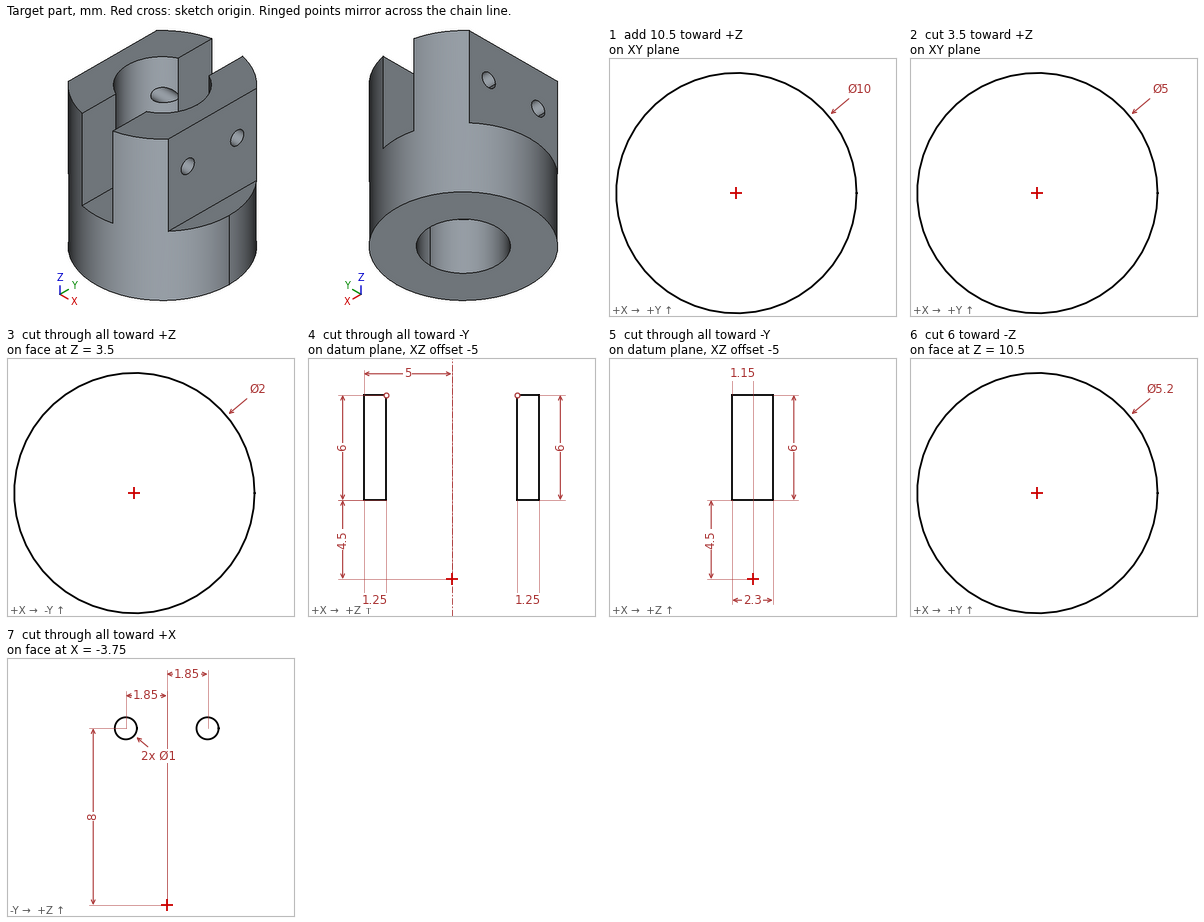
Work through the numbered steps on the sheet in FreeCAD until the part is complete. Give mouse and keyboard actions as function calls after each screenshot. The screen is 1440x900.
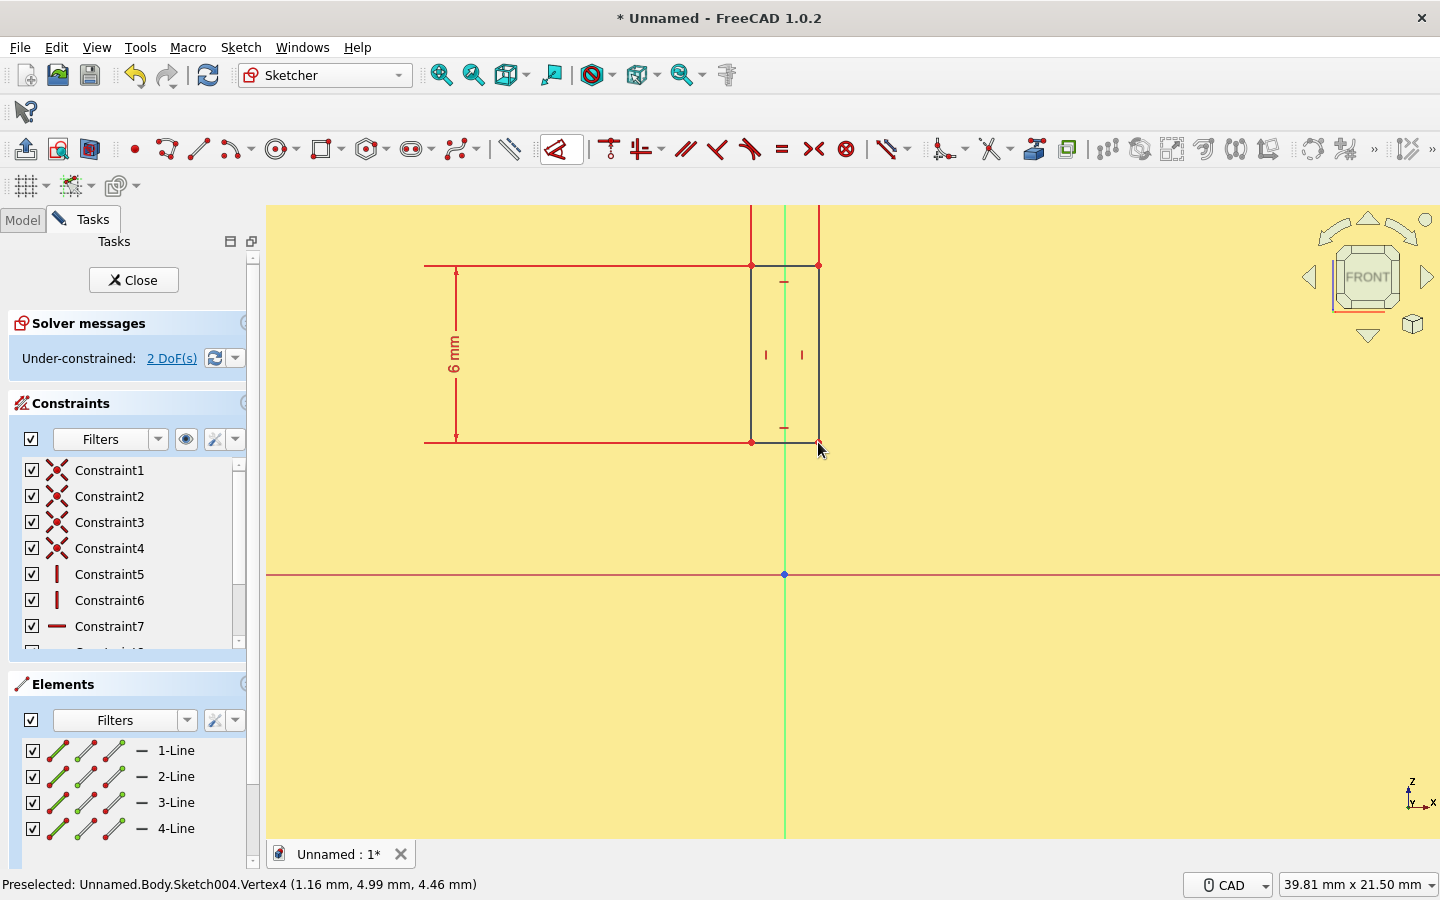
click(751, 443)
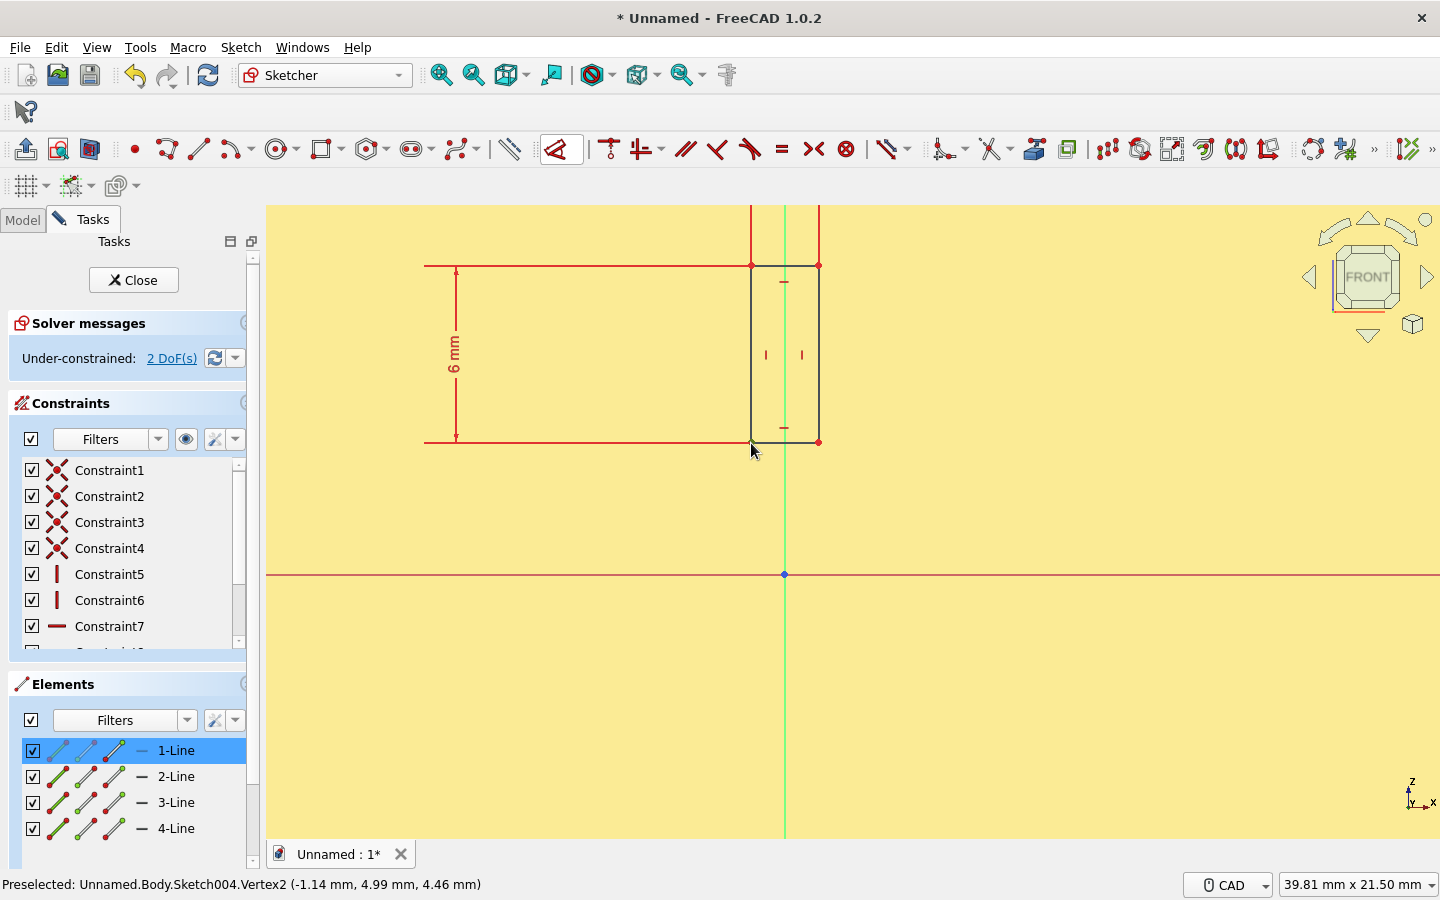
key(i)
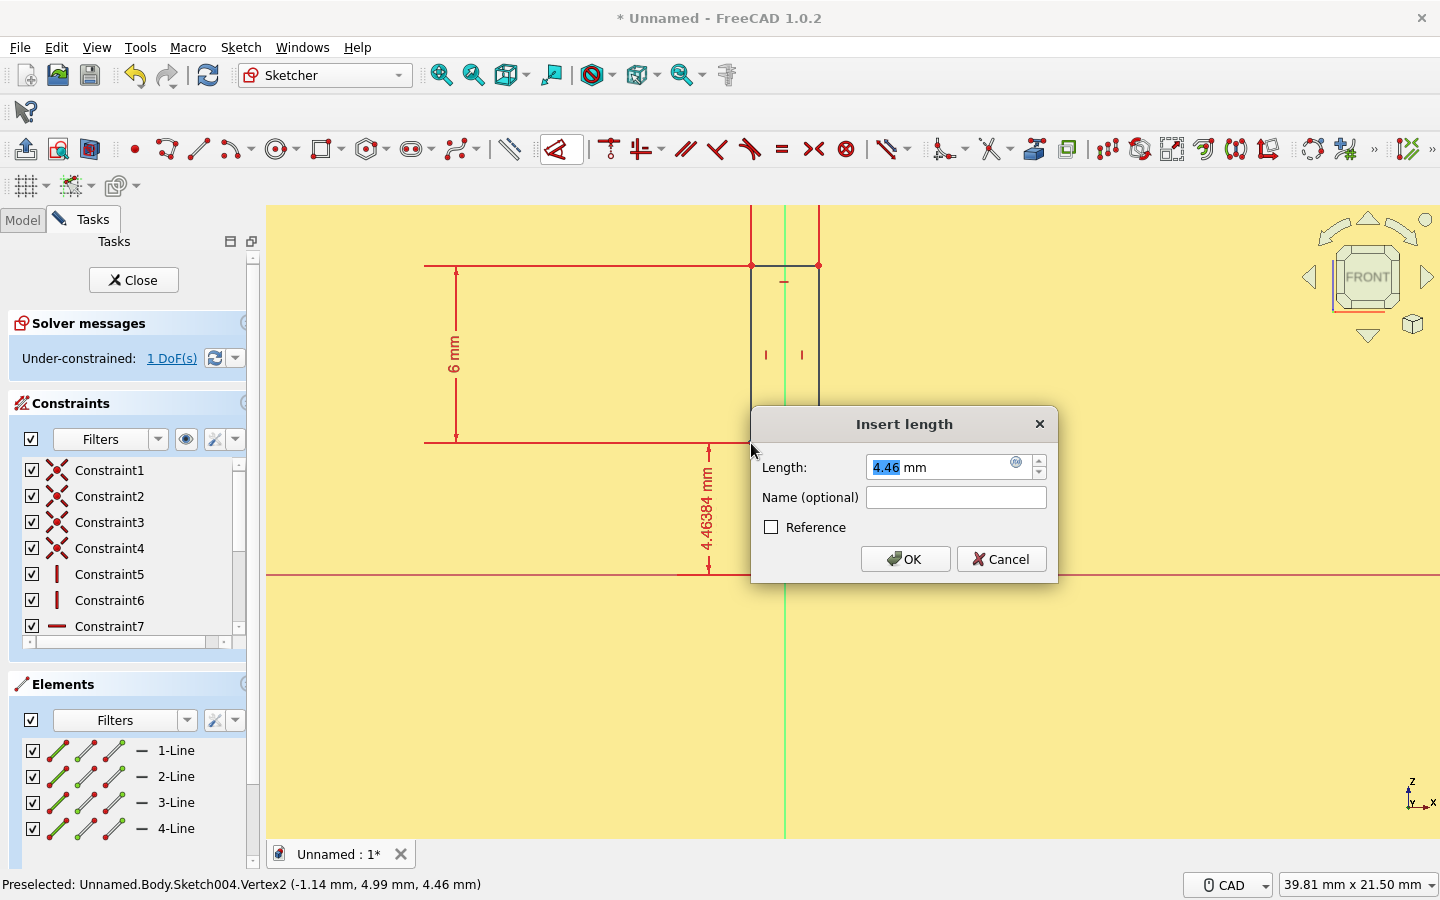
text(4.5)
key(Return)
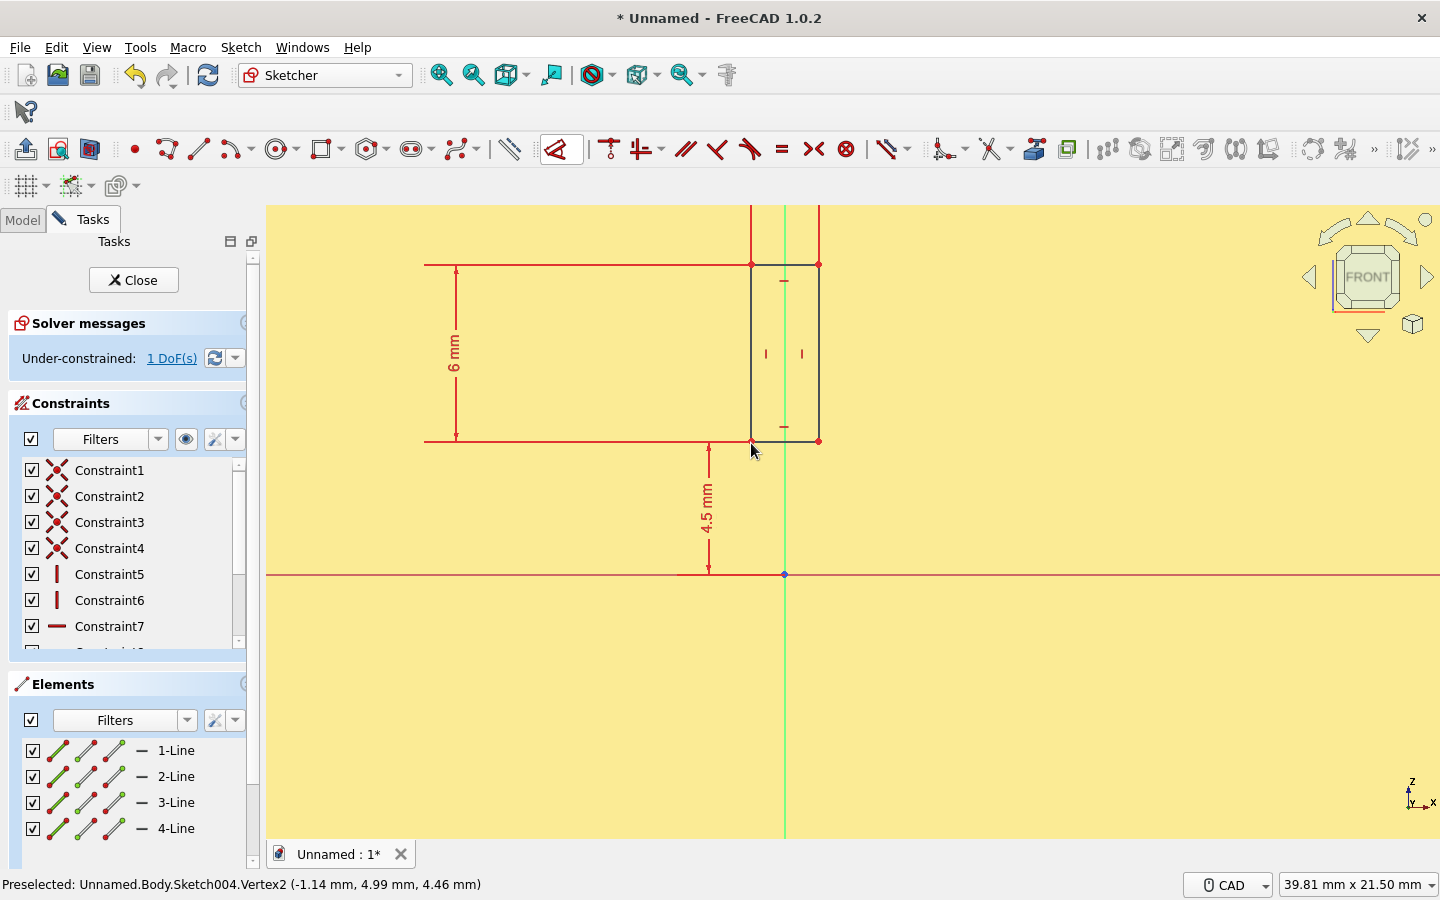
click(751, 265)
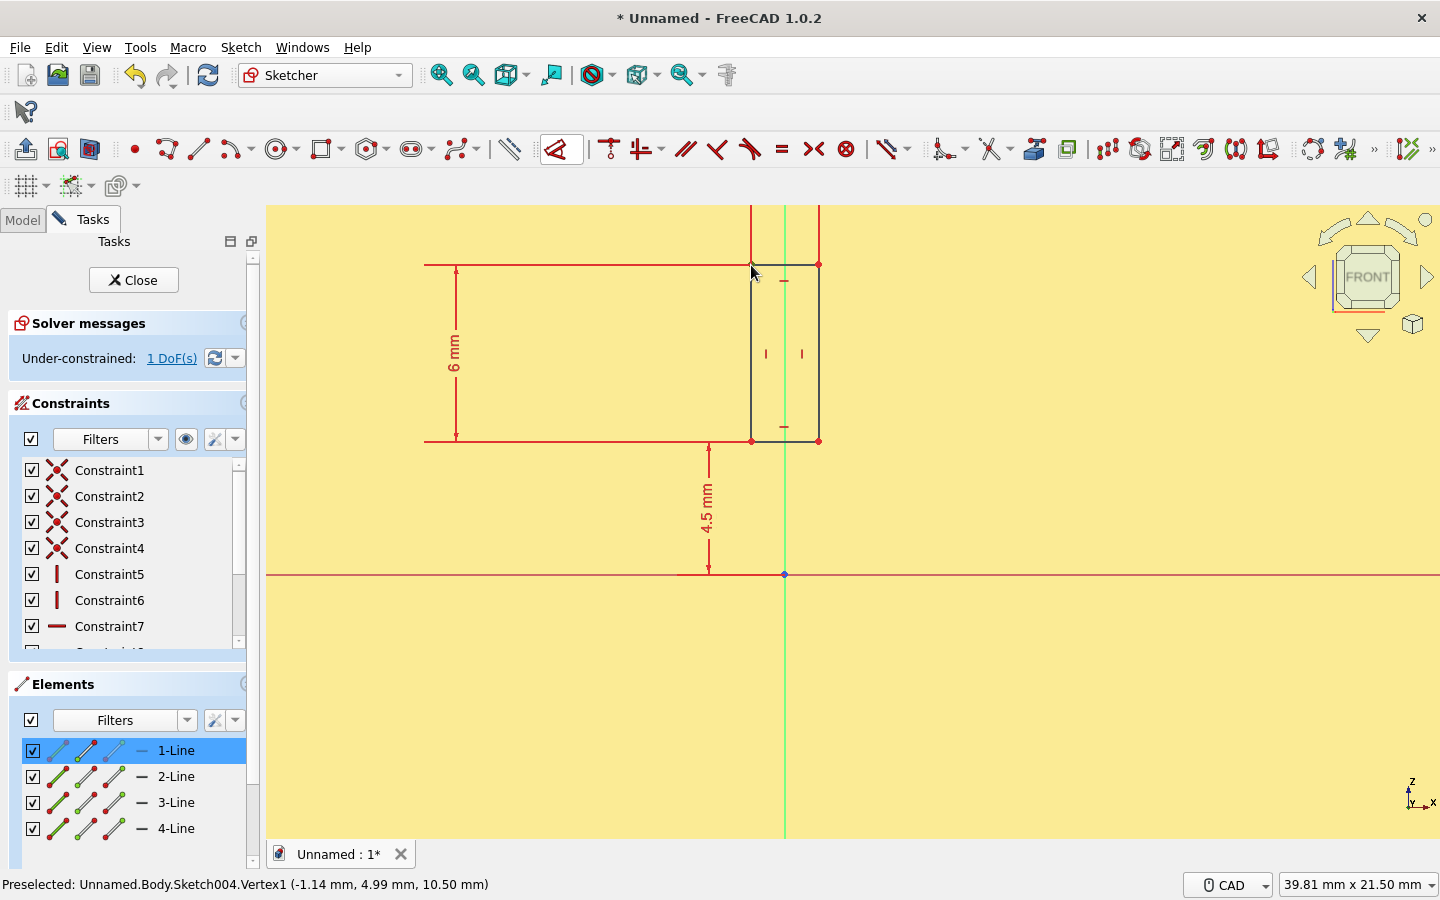
click(578, 150)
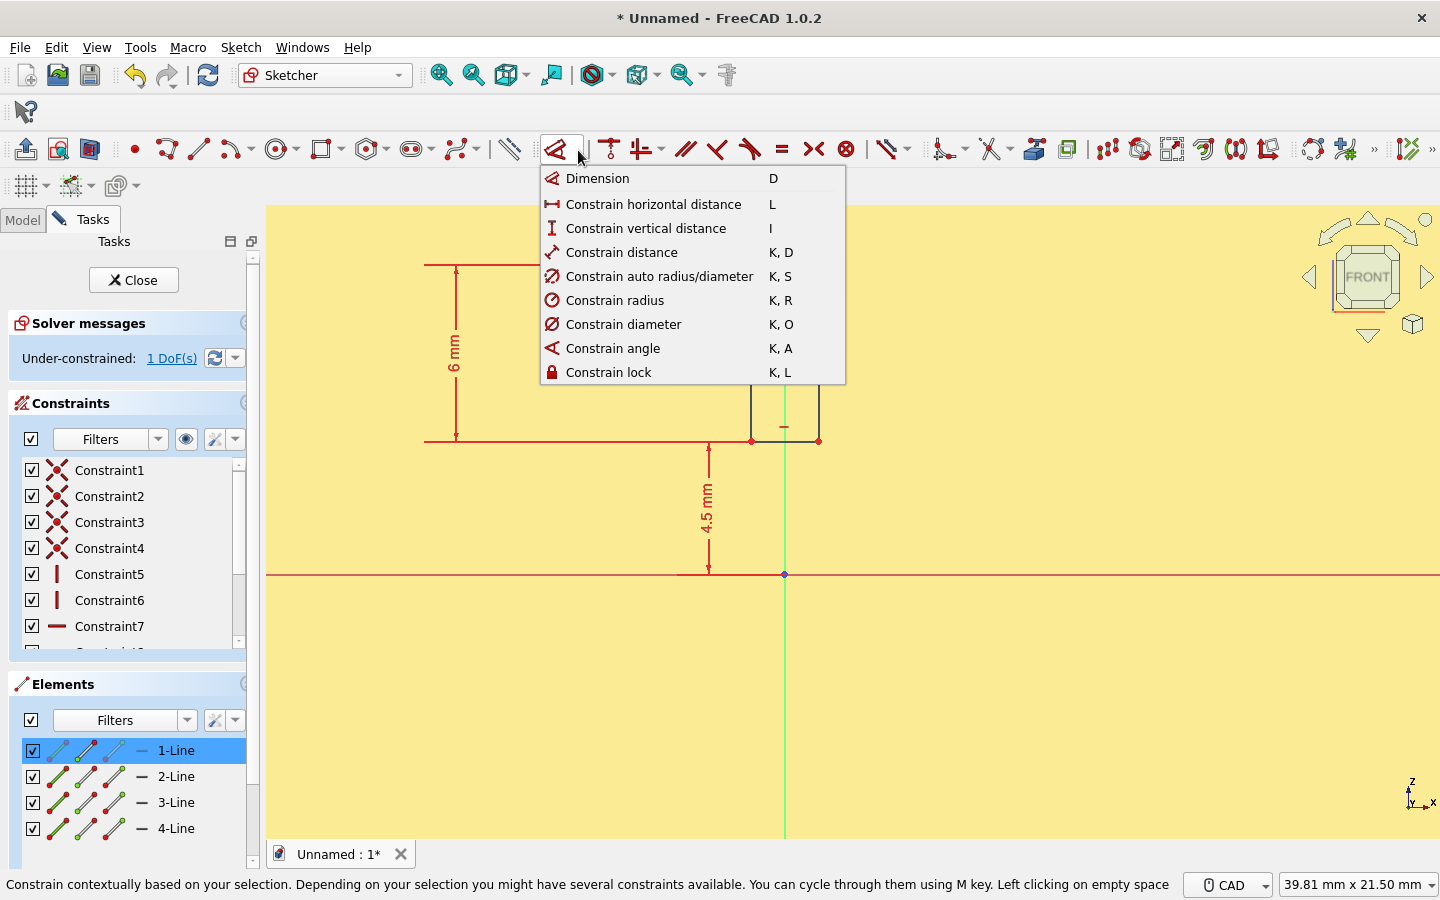
click(693, 204)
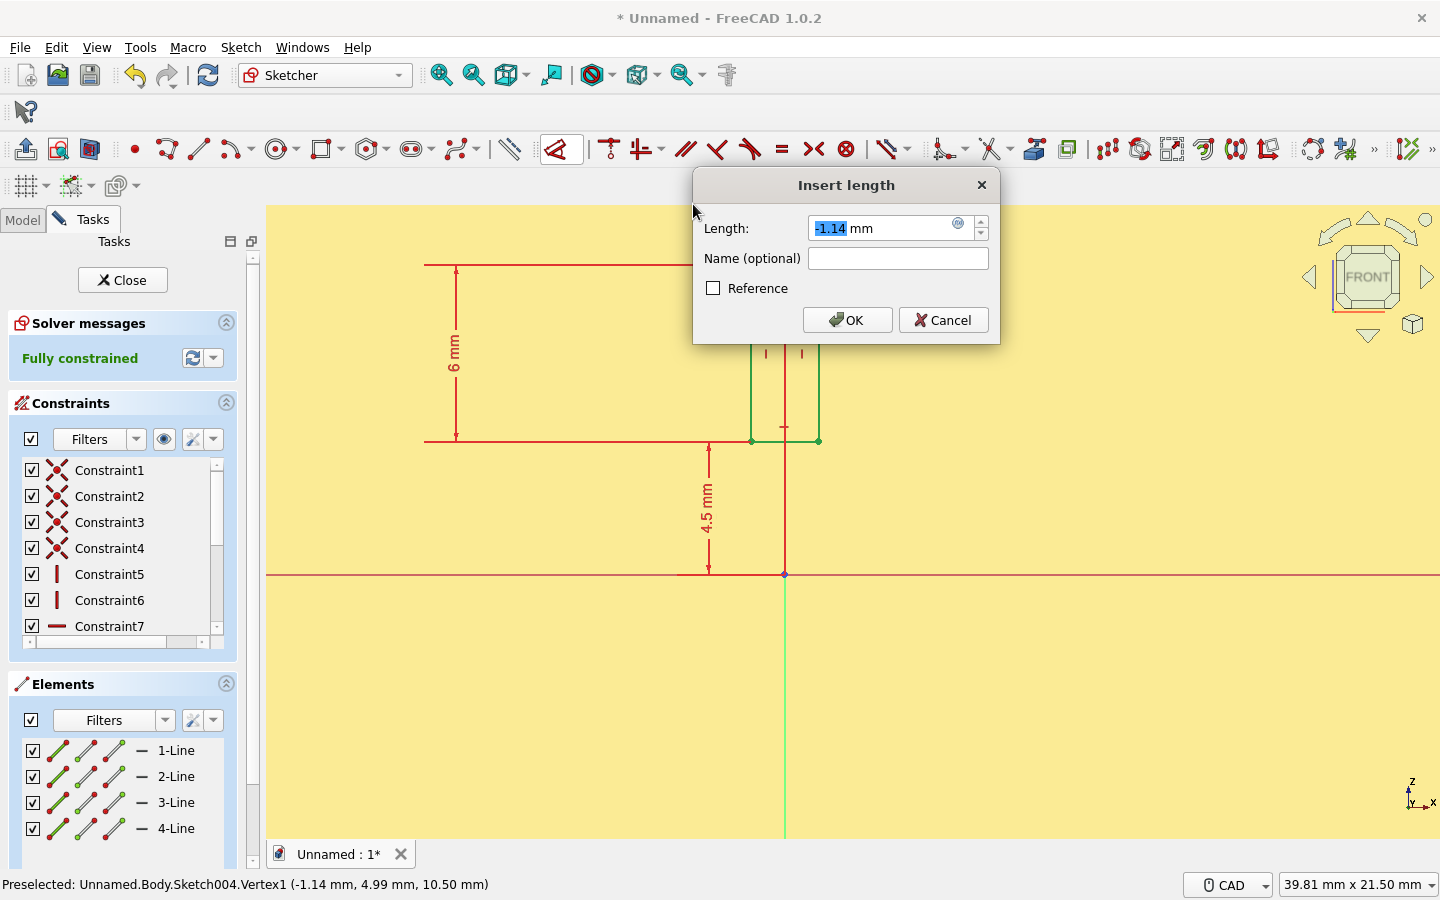
text(-1.15)
key(Return)